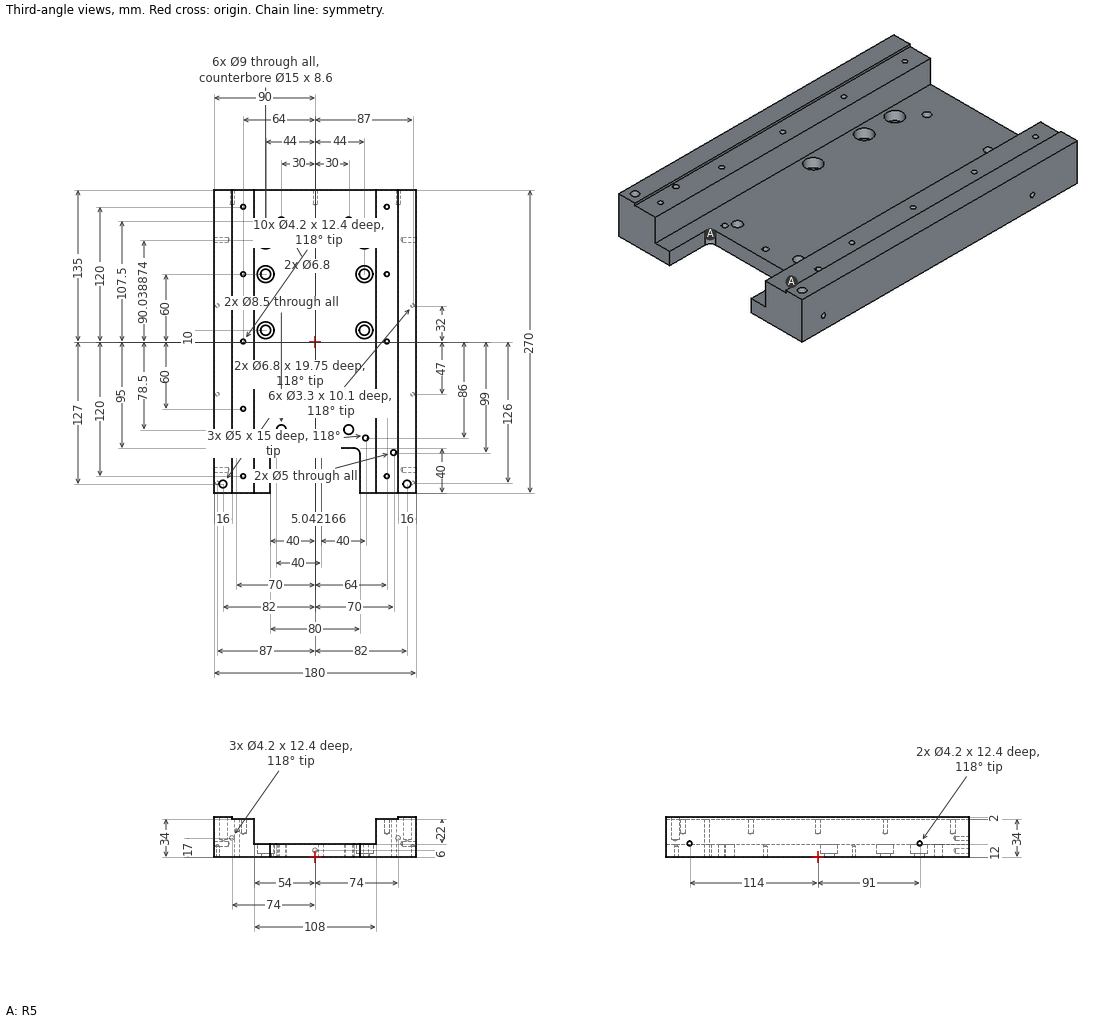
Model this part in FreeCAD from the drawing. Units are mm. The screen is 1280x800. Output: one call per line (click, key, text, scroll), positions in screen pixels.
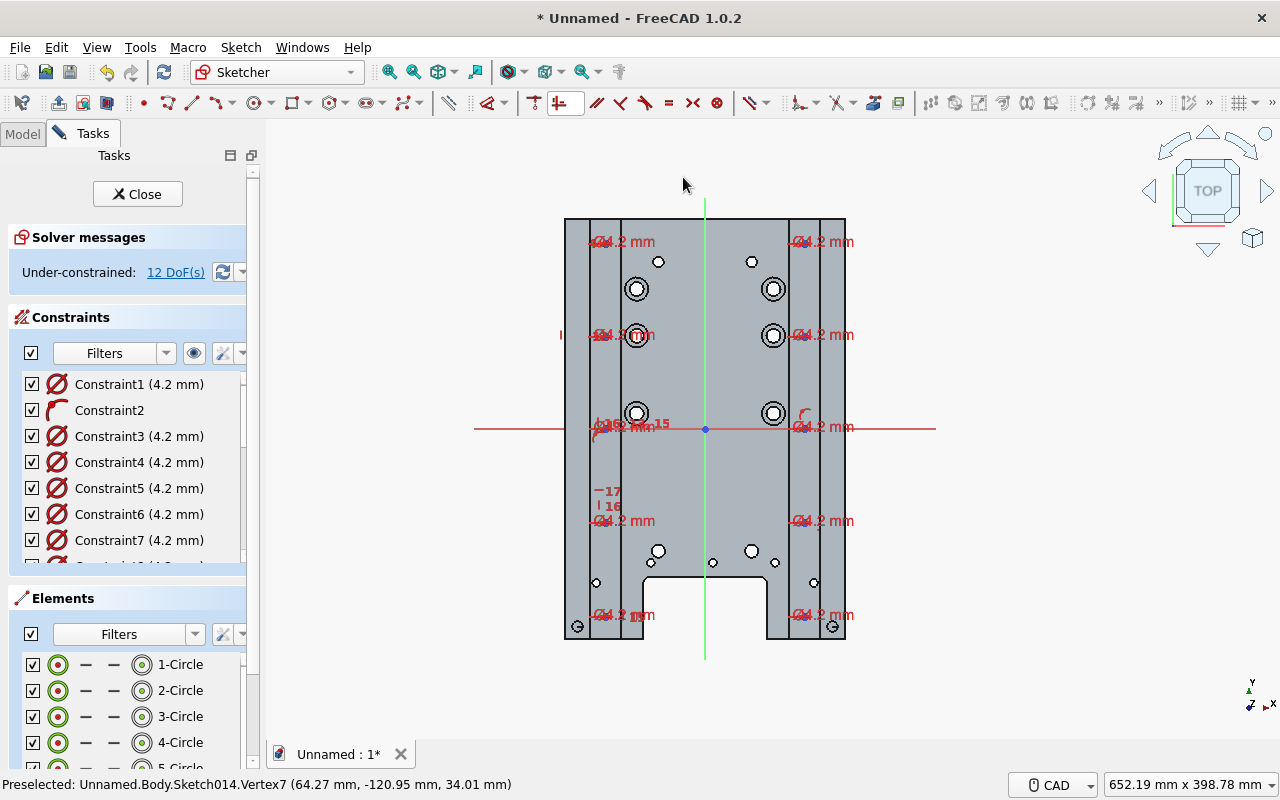
click(606, 617)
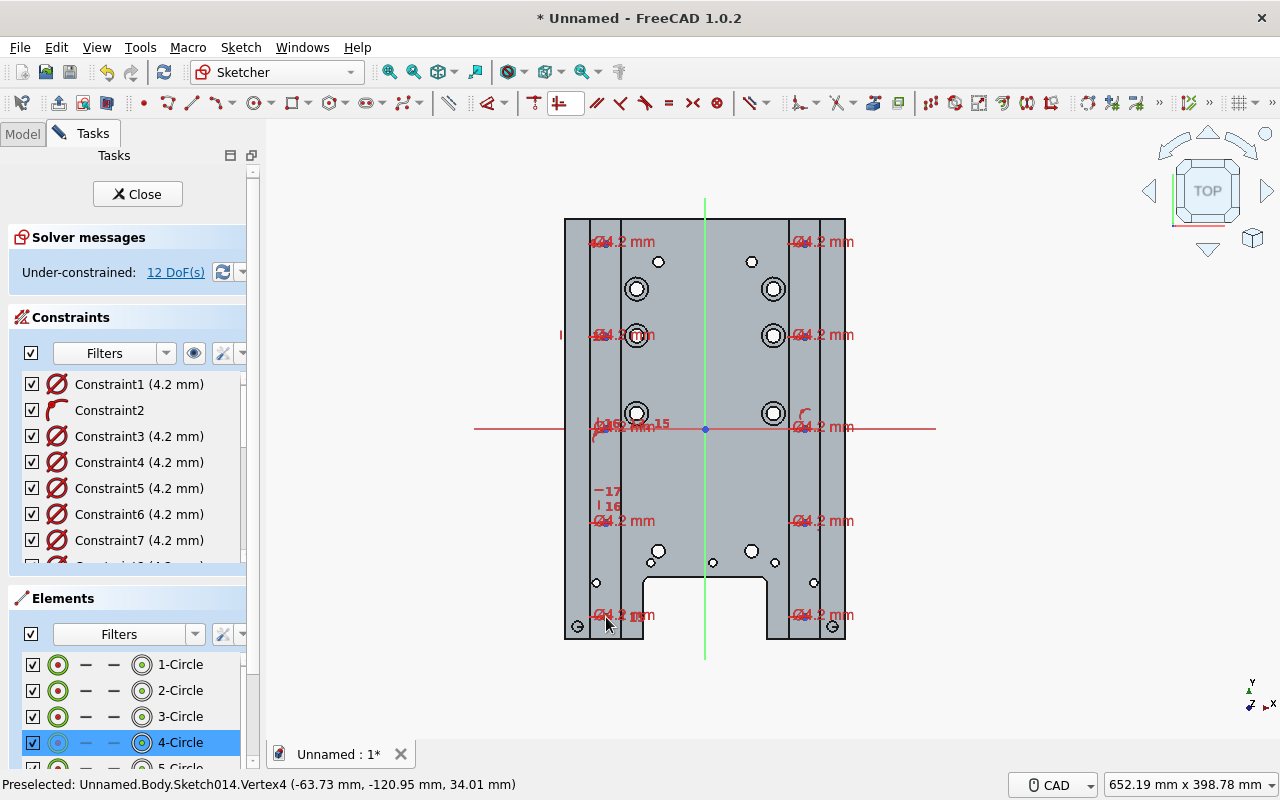
click(805, 617)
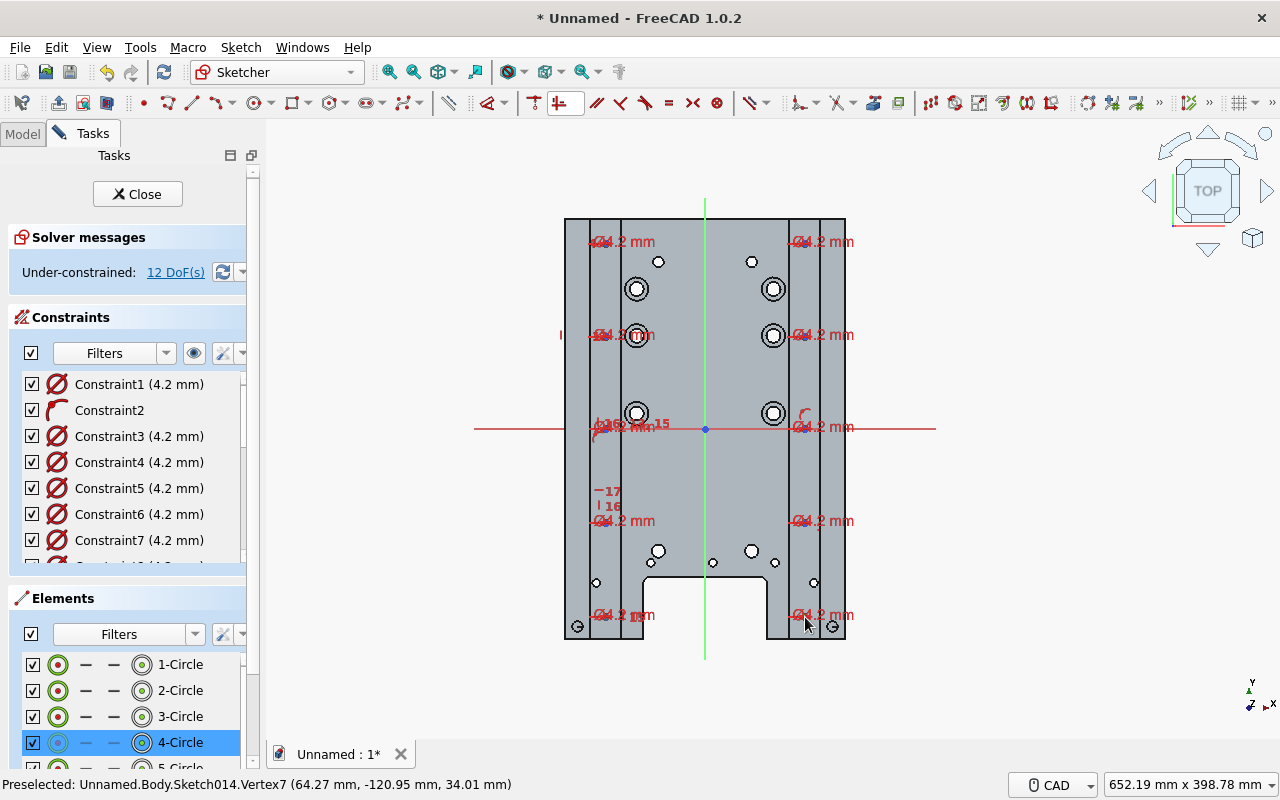
click(578, 104)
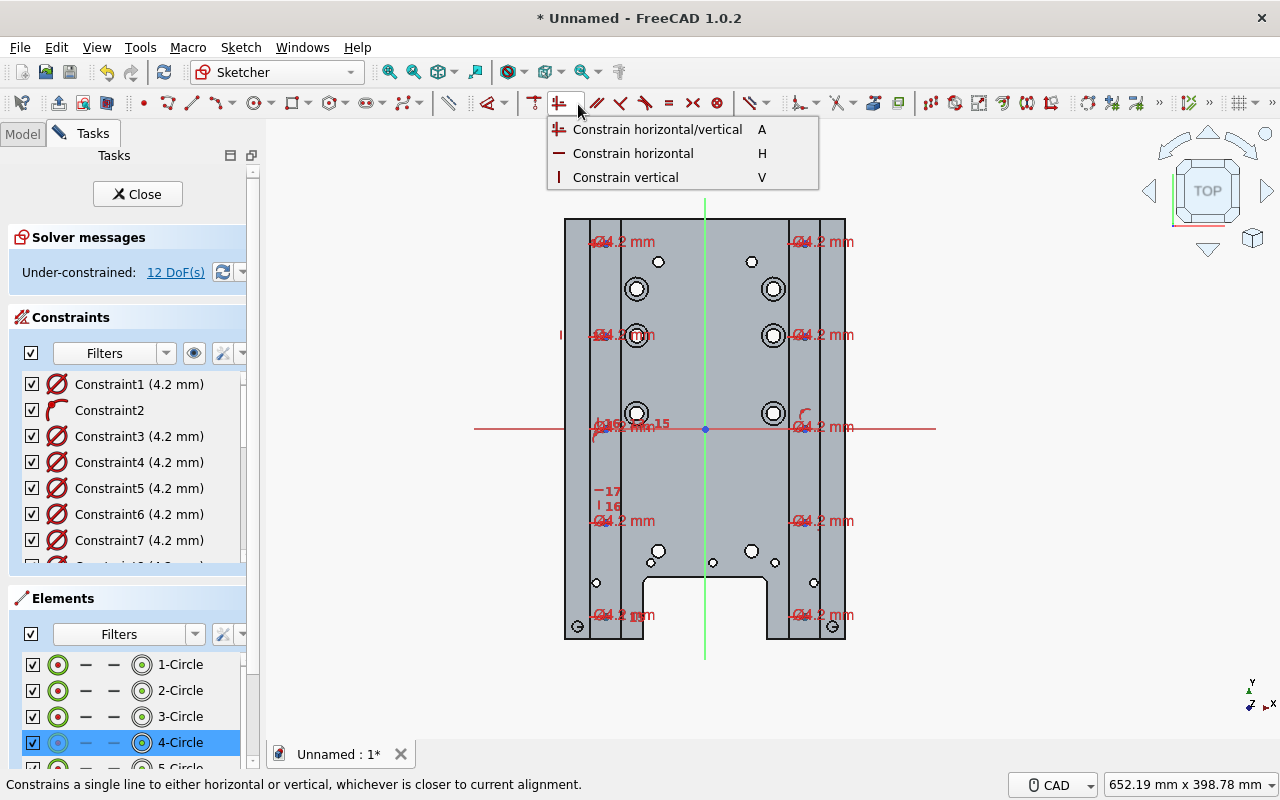
click(683, 153)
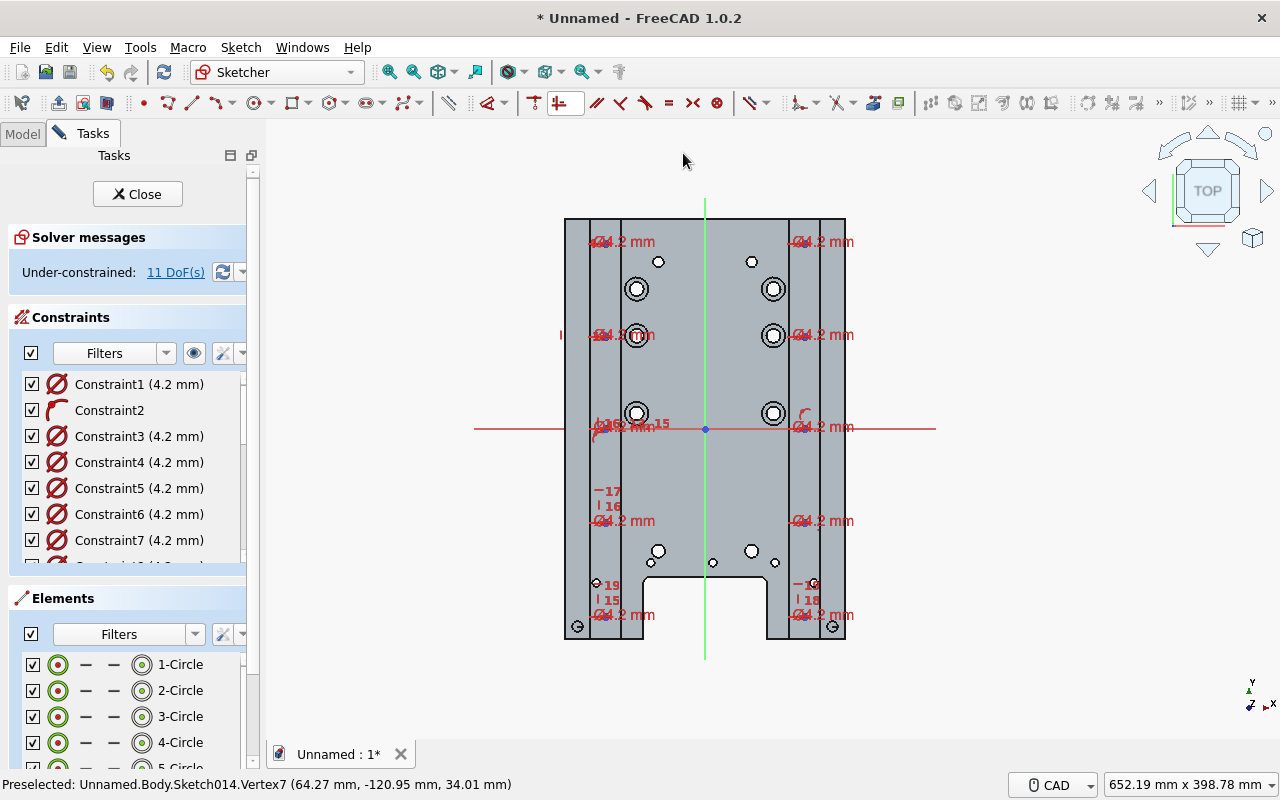
click(805, 523)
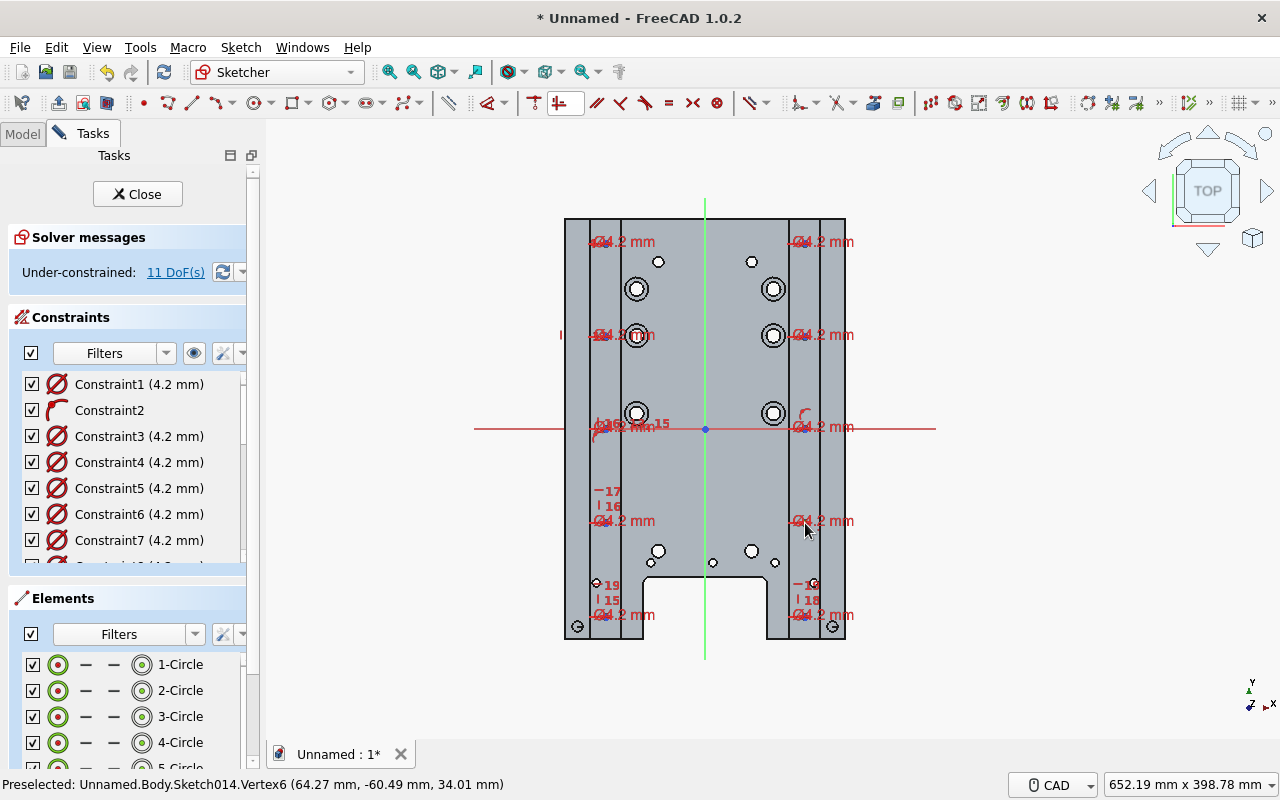
click(805, 244)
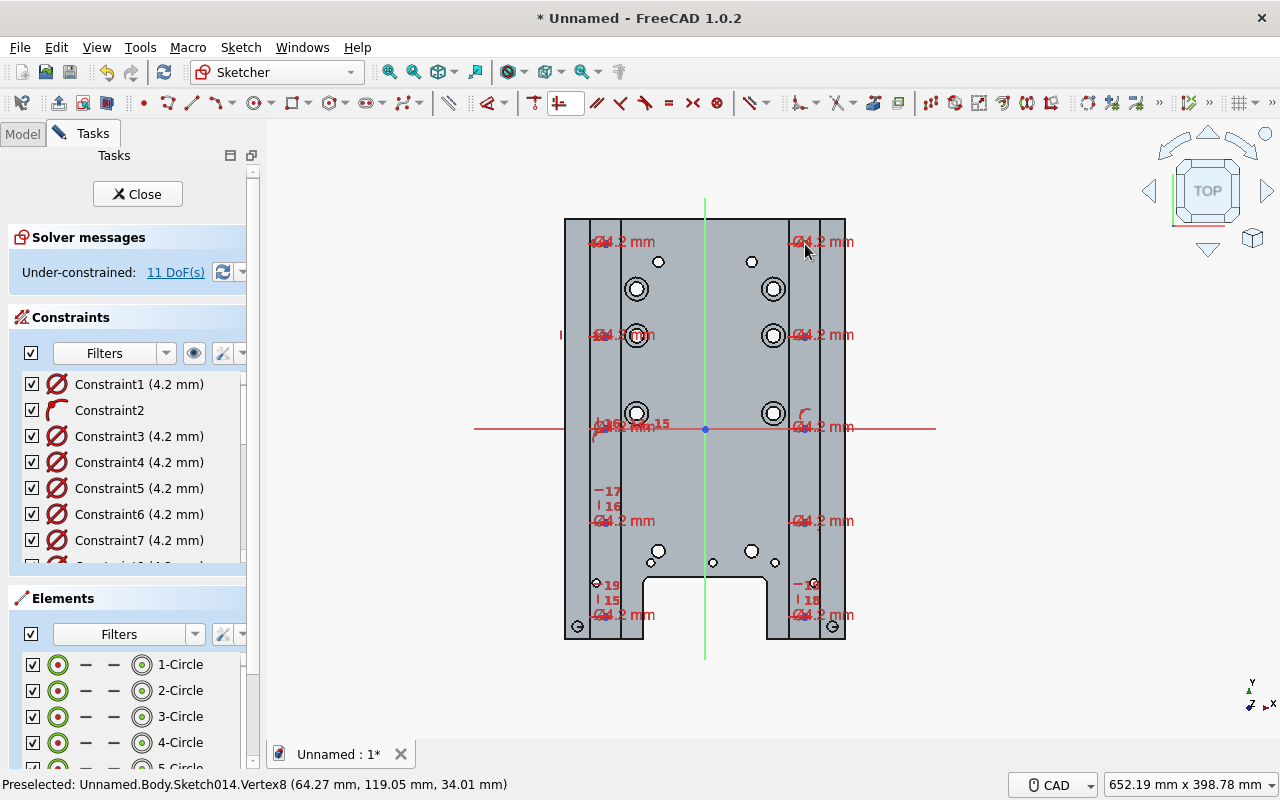
key(v)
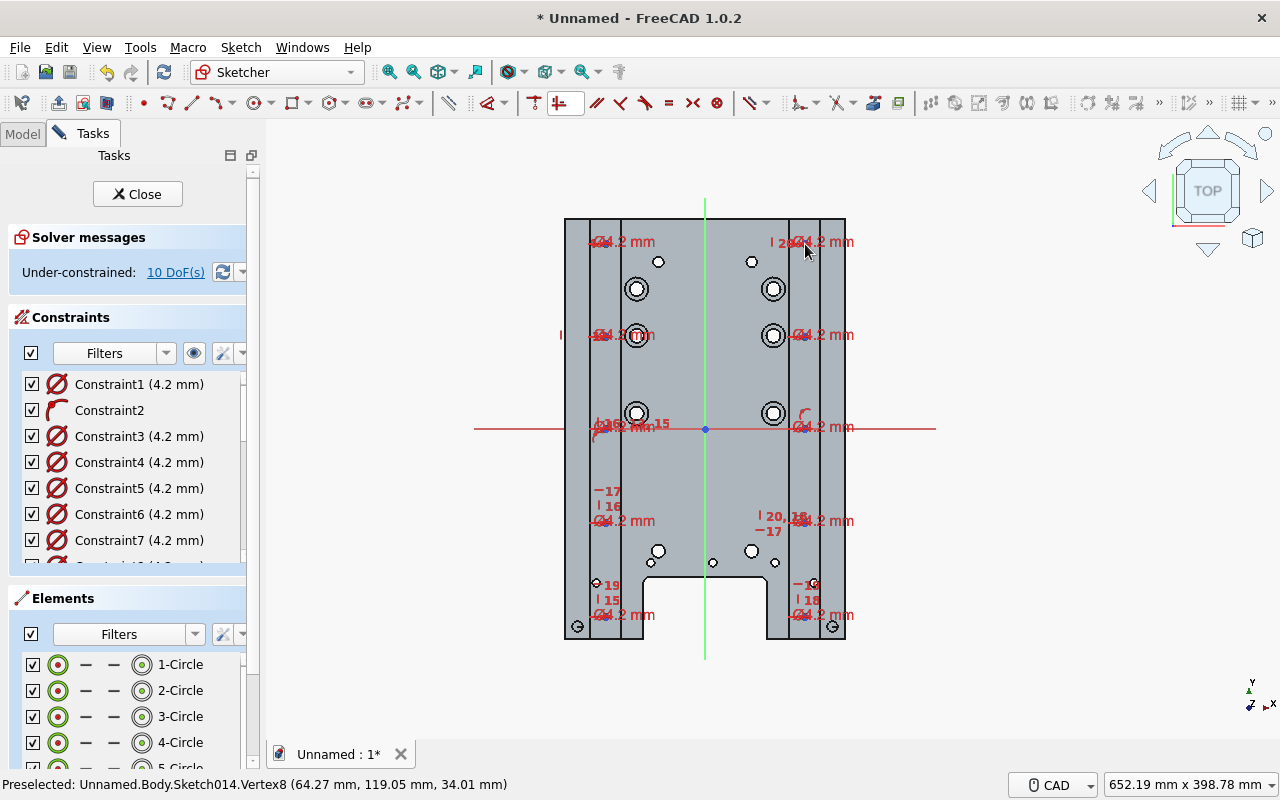
click(606, 244)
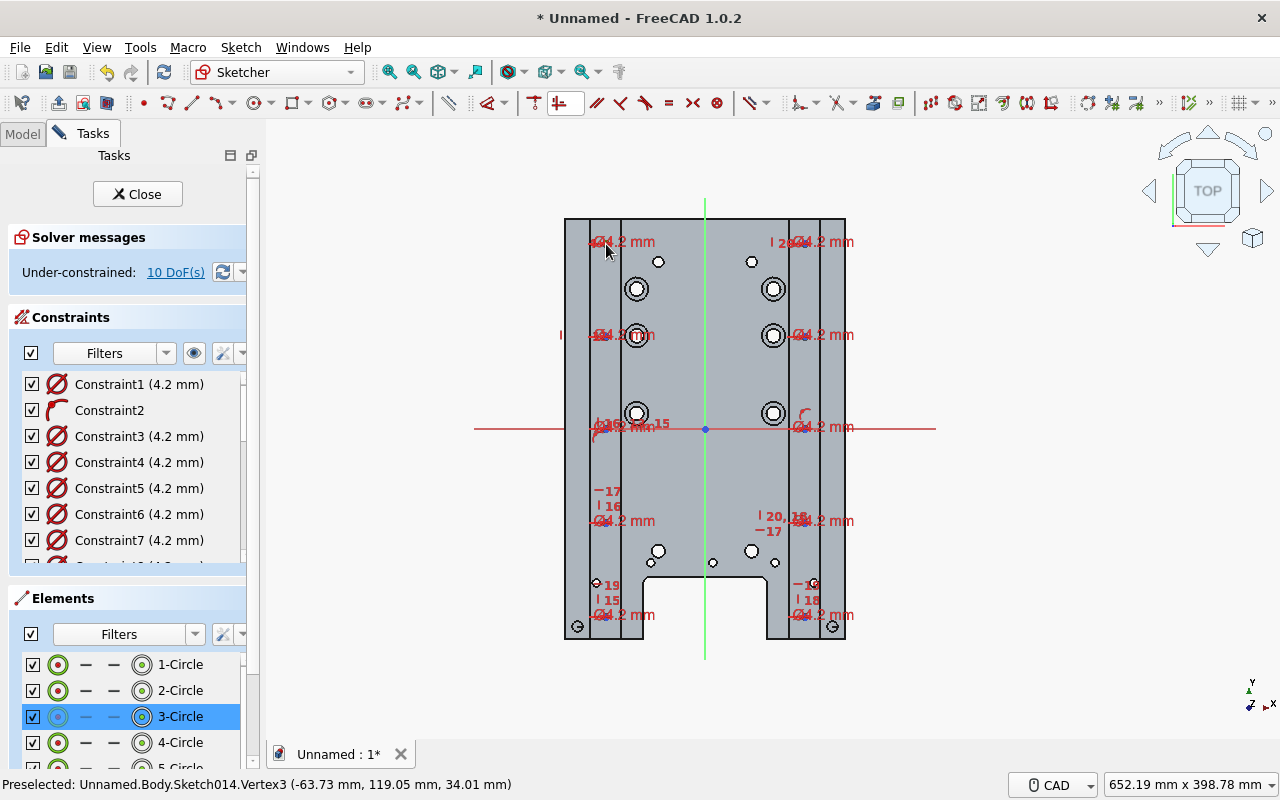
click(805, 244)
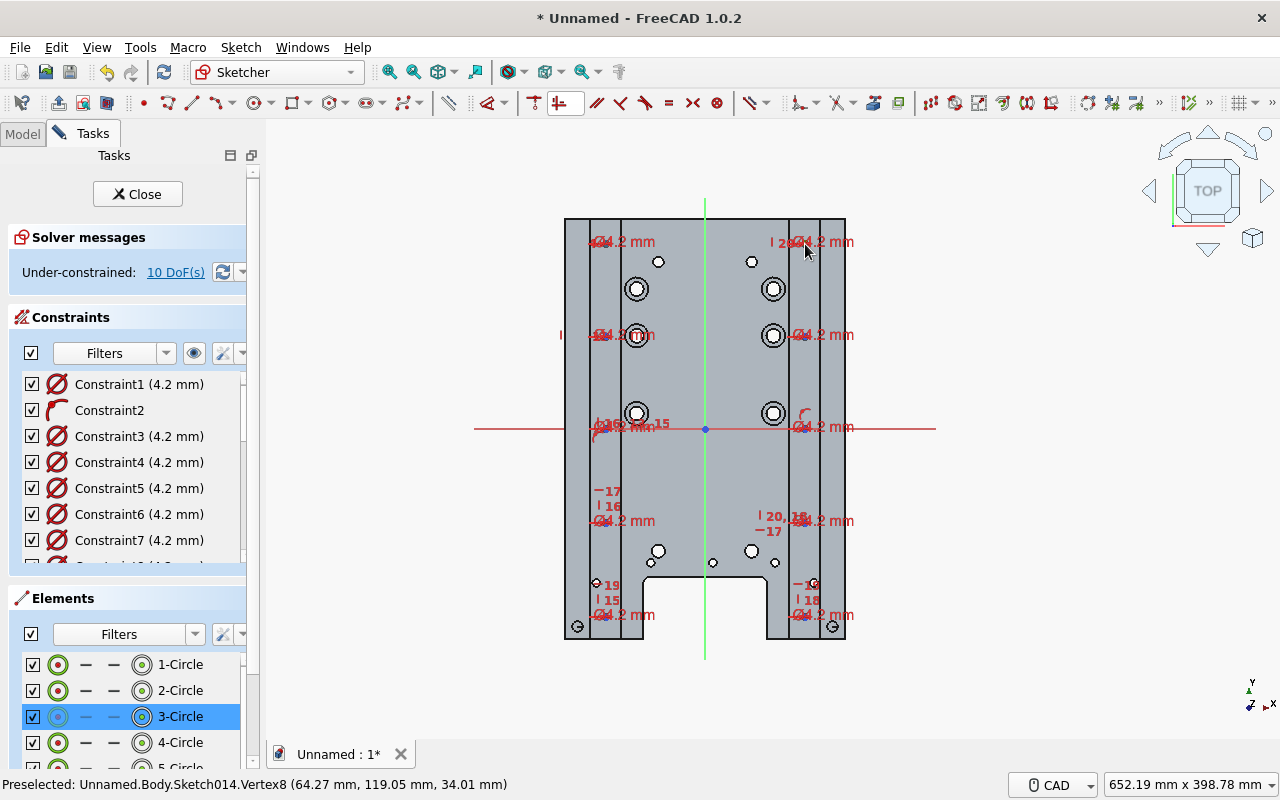
key(h)